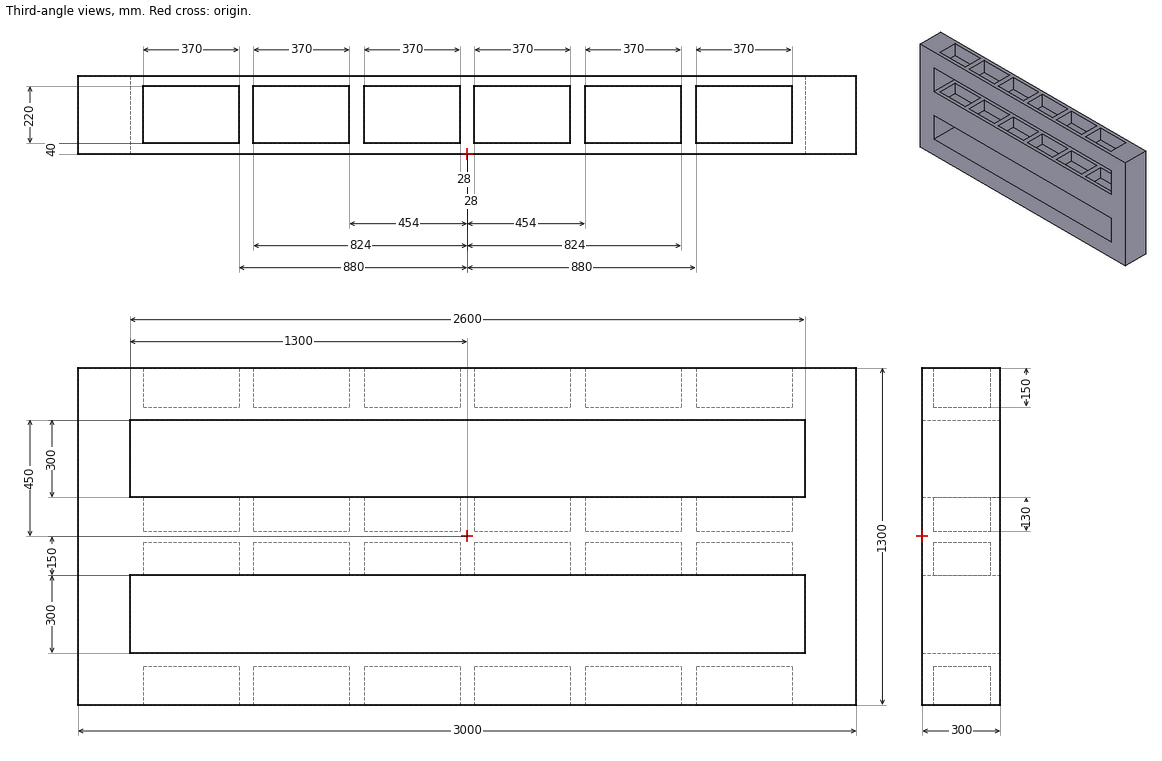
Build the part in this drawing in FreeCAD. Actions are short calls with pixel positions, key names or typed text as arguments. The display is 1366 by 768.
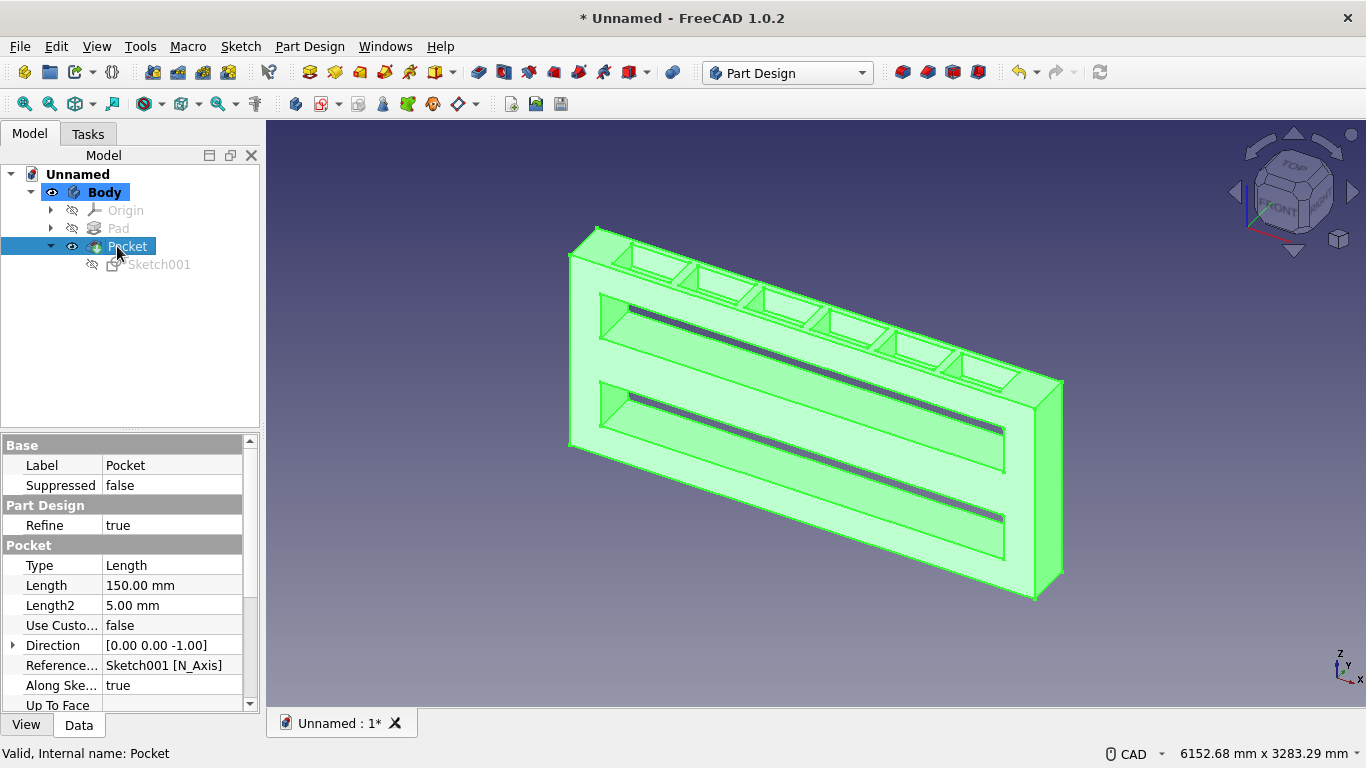
click(153, 72)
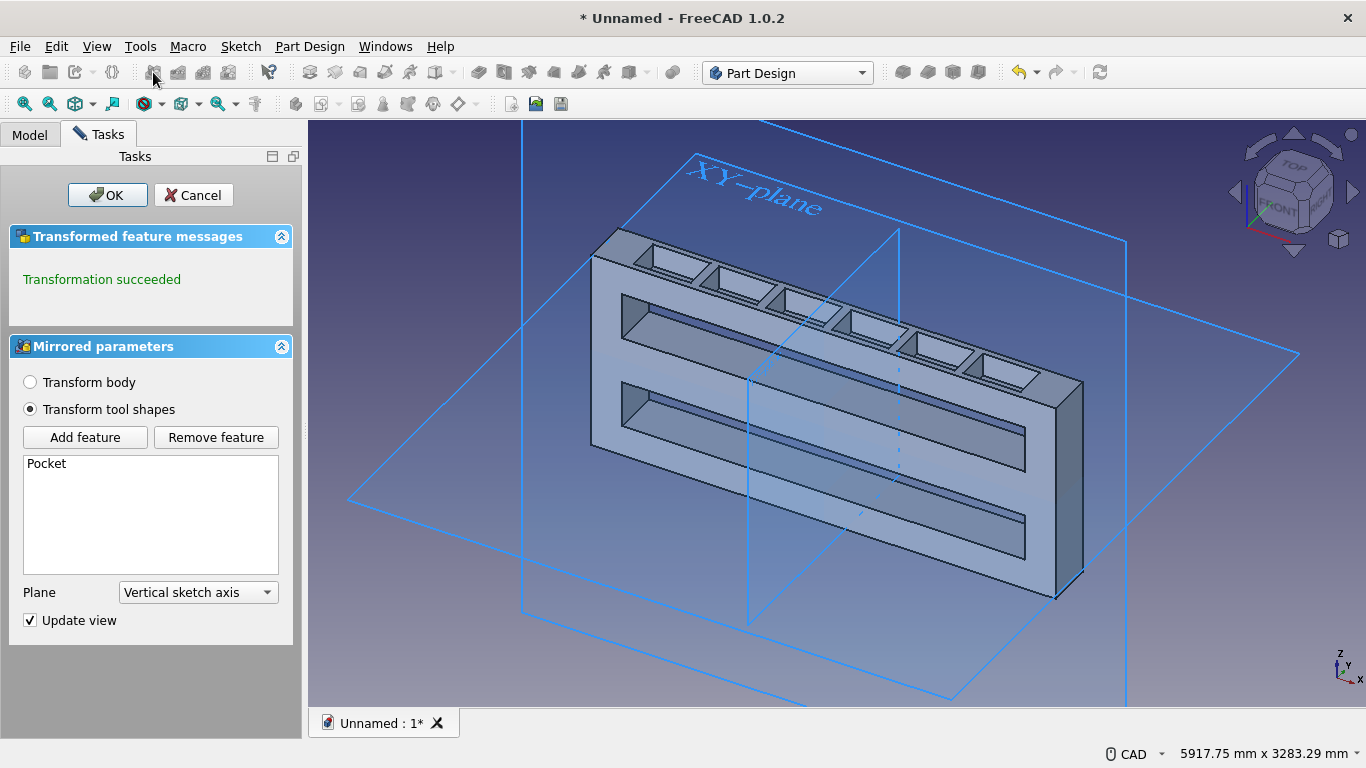
click(199, 592)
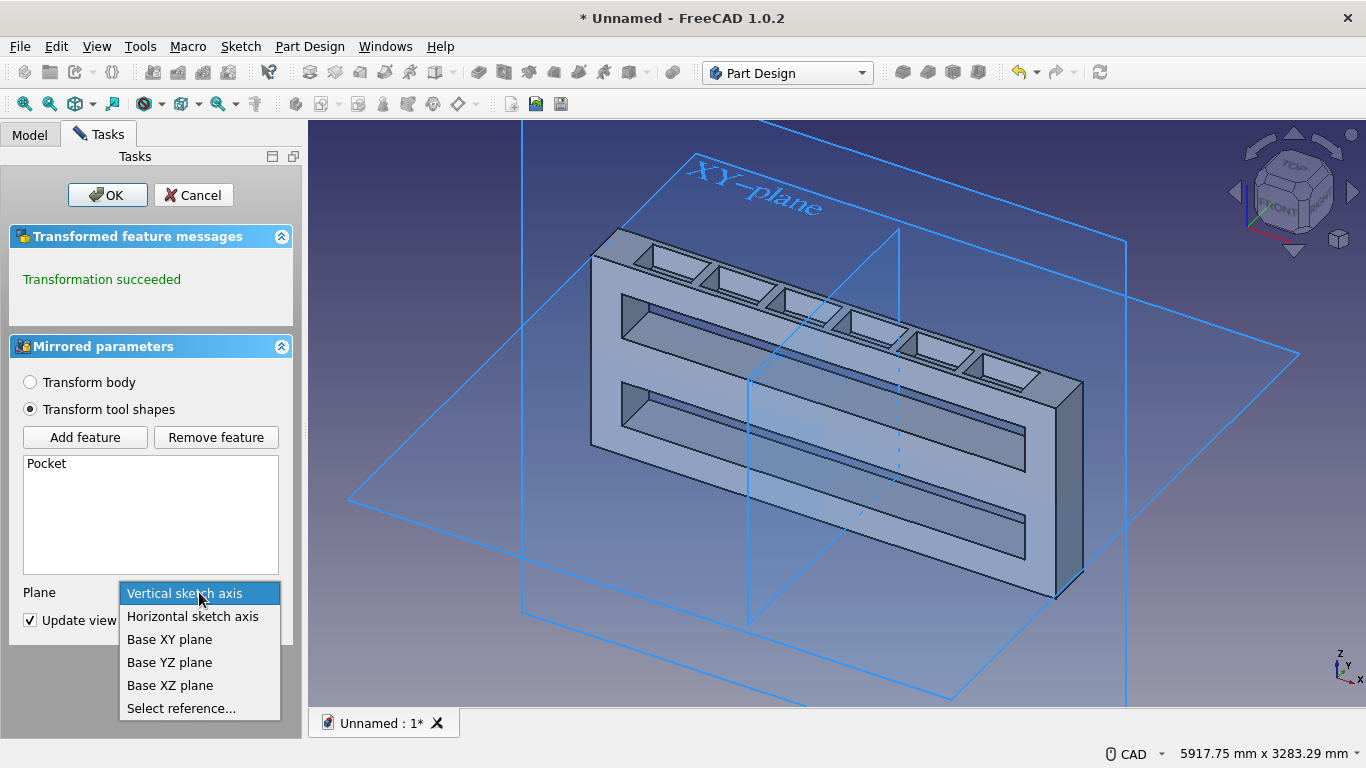
click(198, 640)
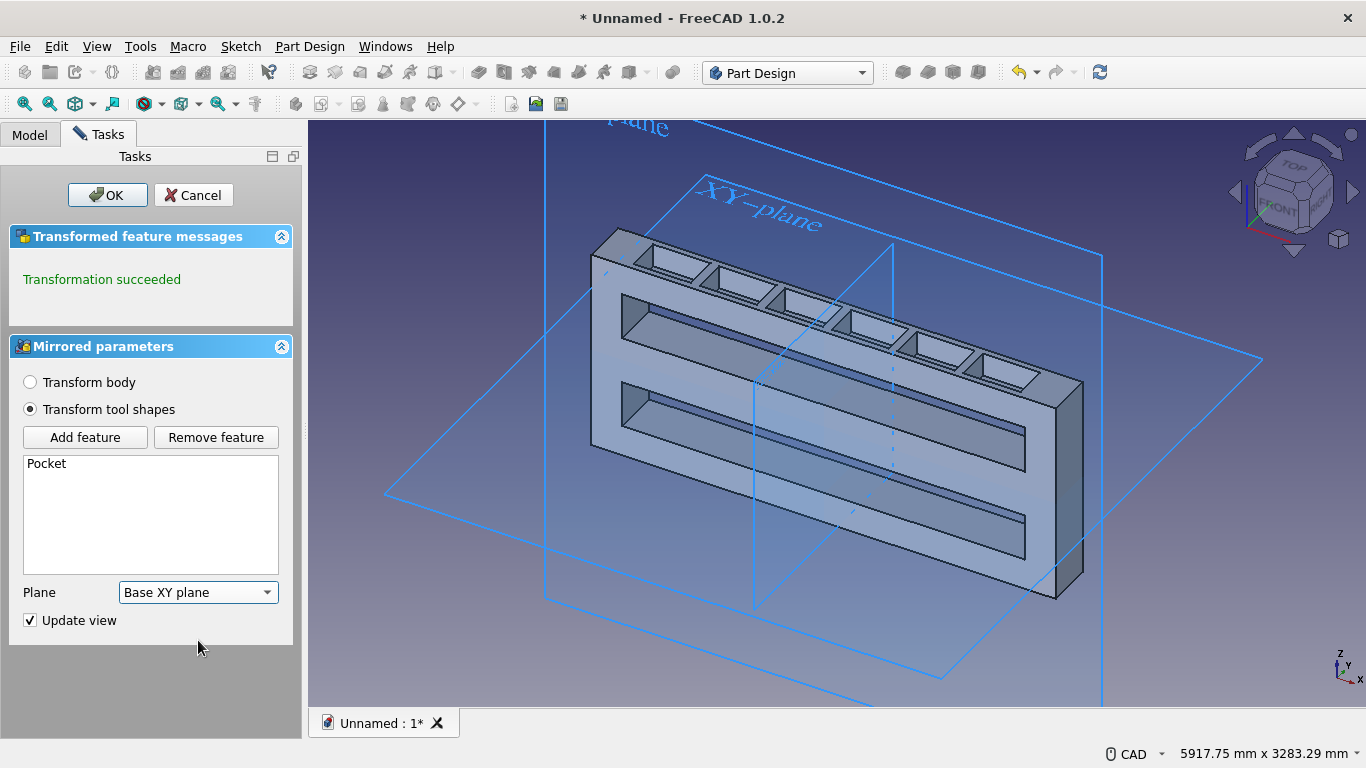
click(108, 195)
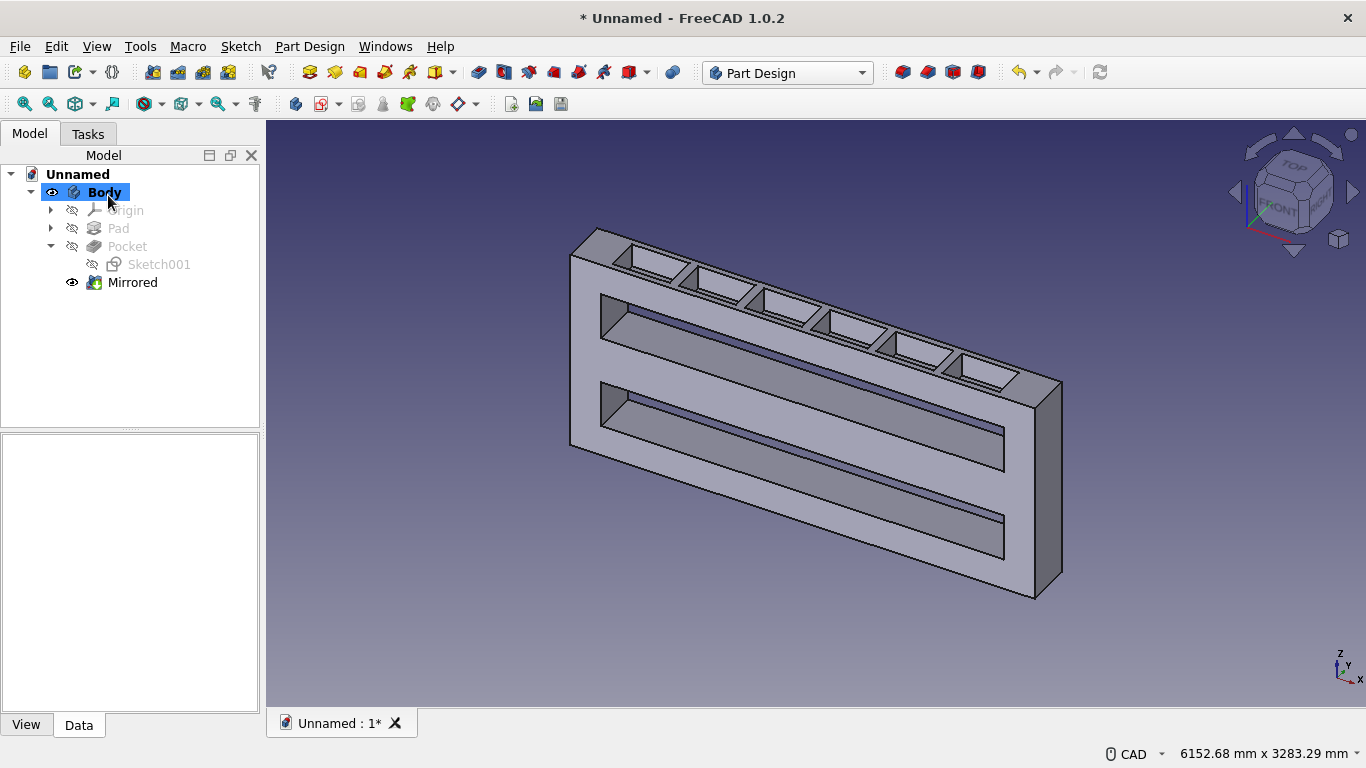
click(51, 210)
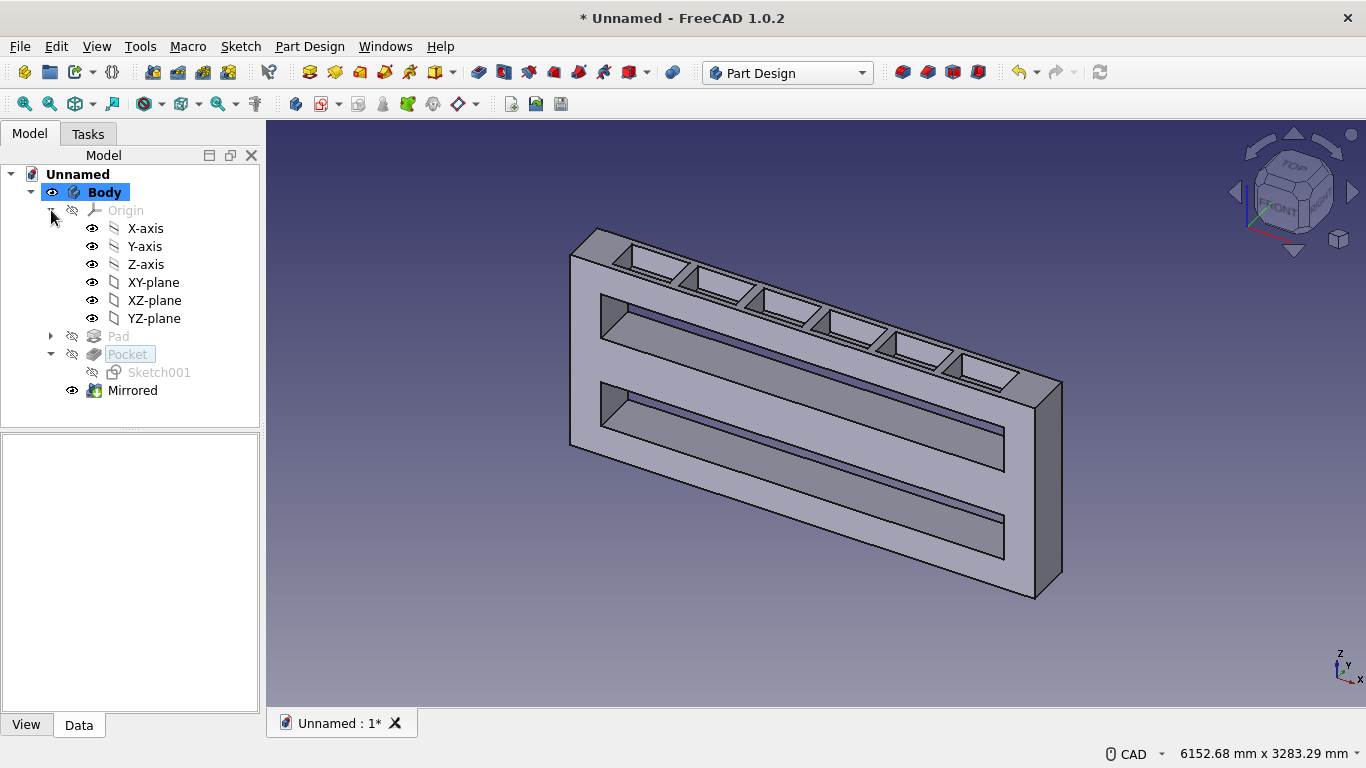
click(137, 282)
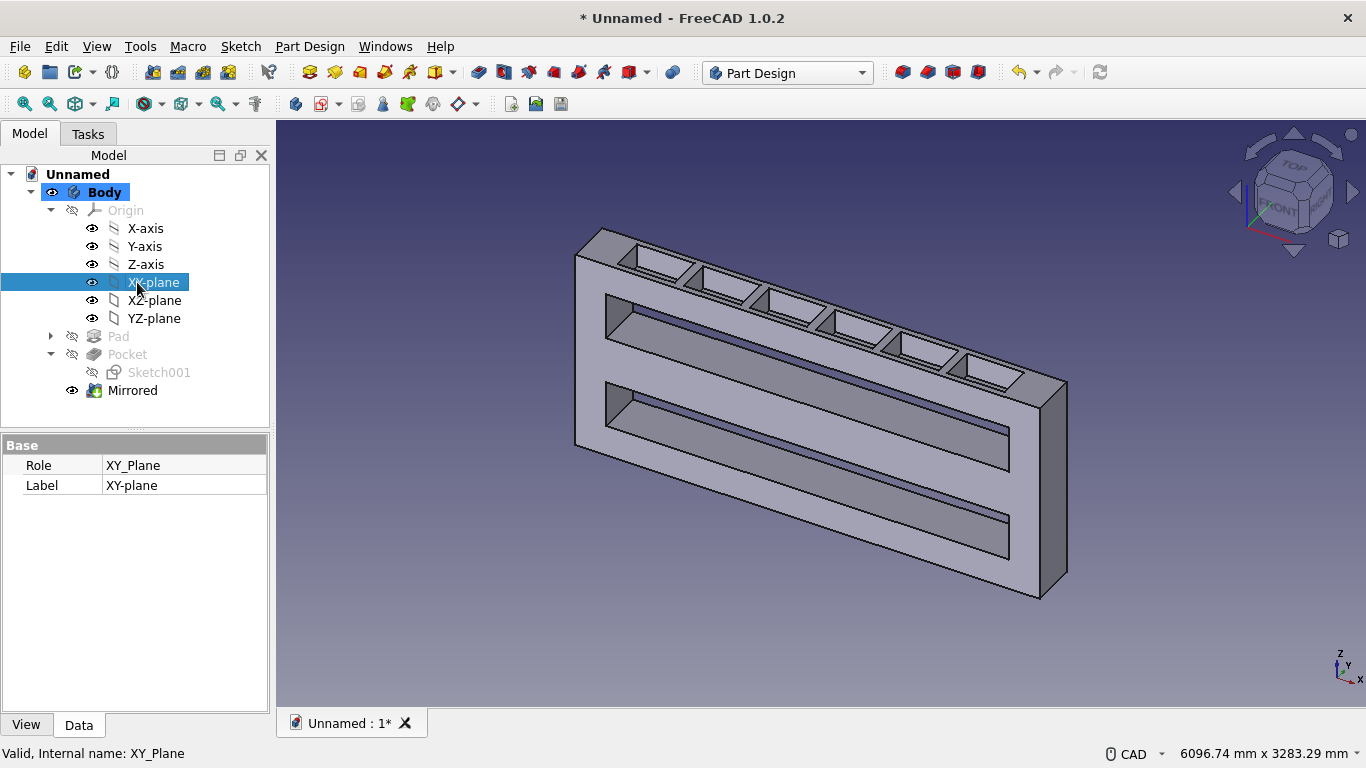
click(458, 104)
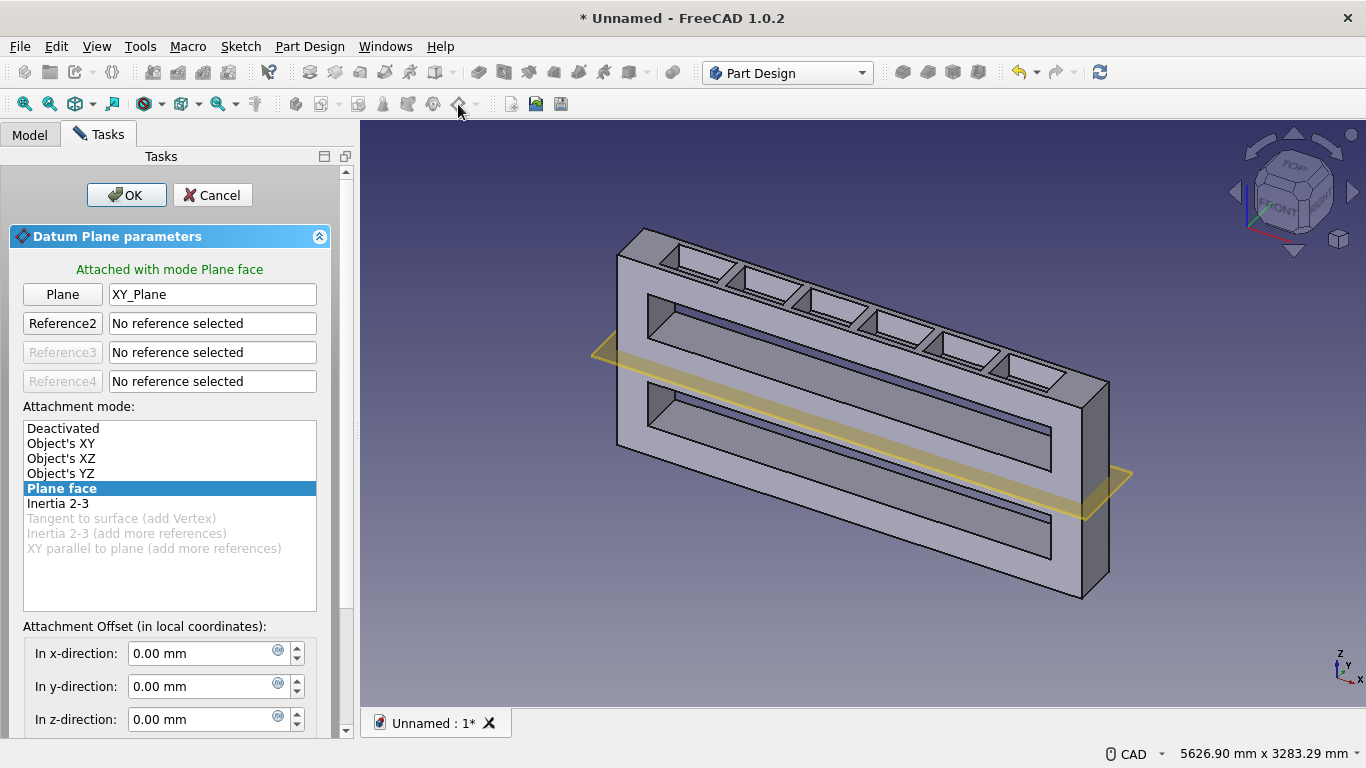
triple_click(210, 720)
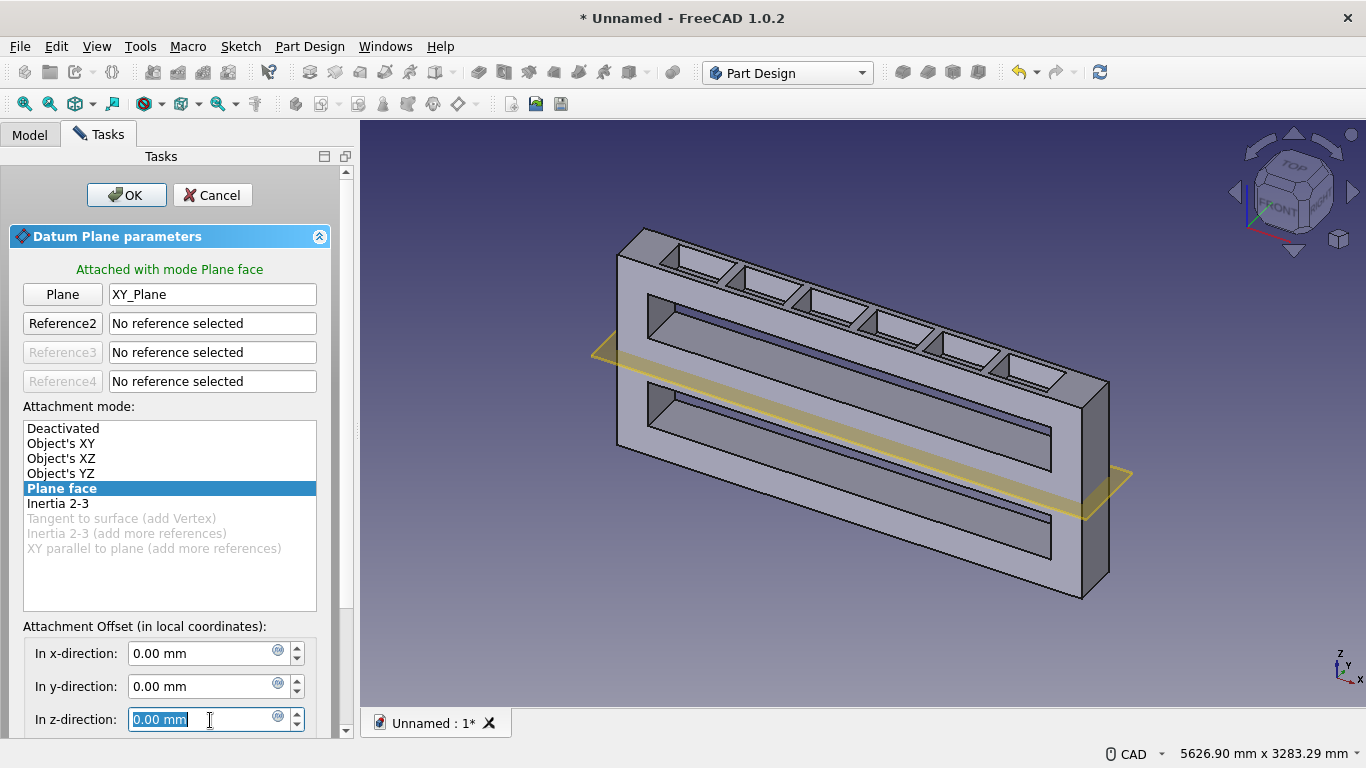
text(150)
key(Tab)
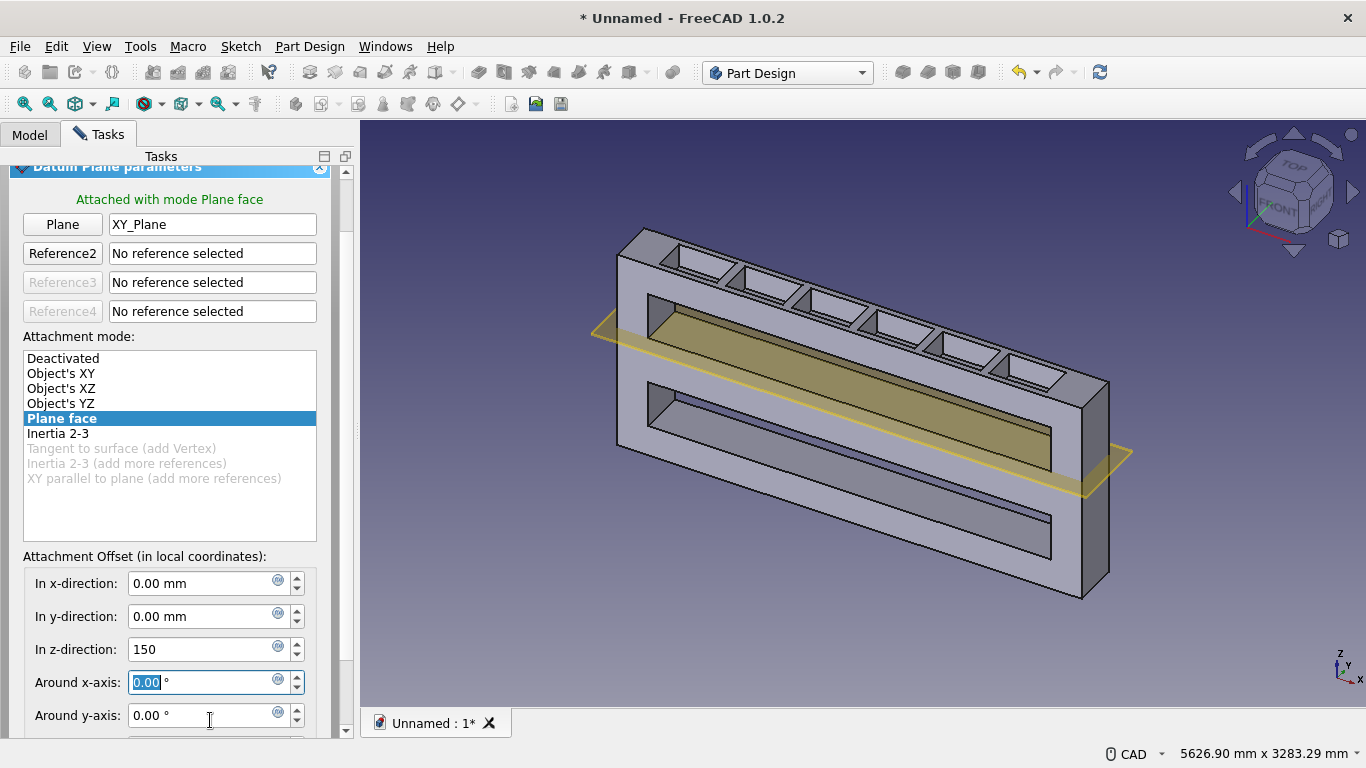
scroll(346, 452, up, 2)